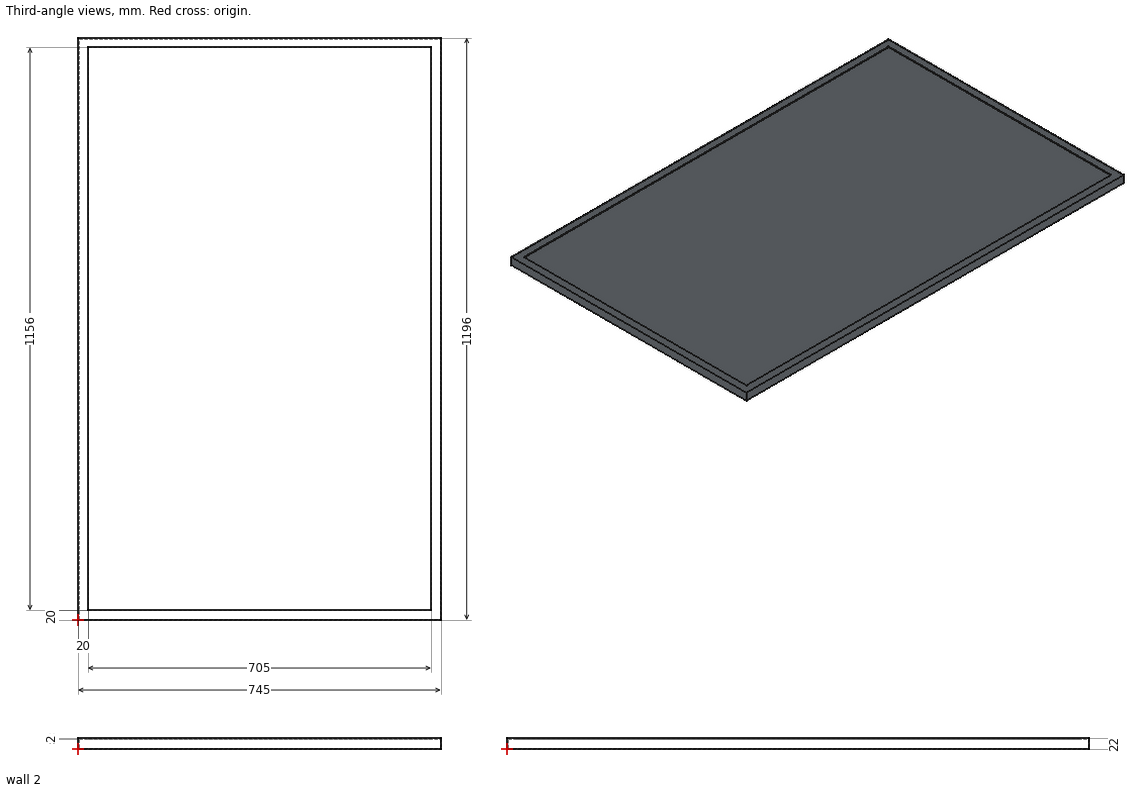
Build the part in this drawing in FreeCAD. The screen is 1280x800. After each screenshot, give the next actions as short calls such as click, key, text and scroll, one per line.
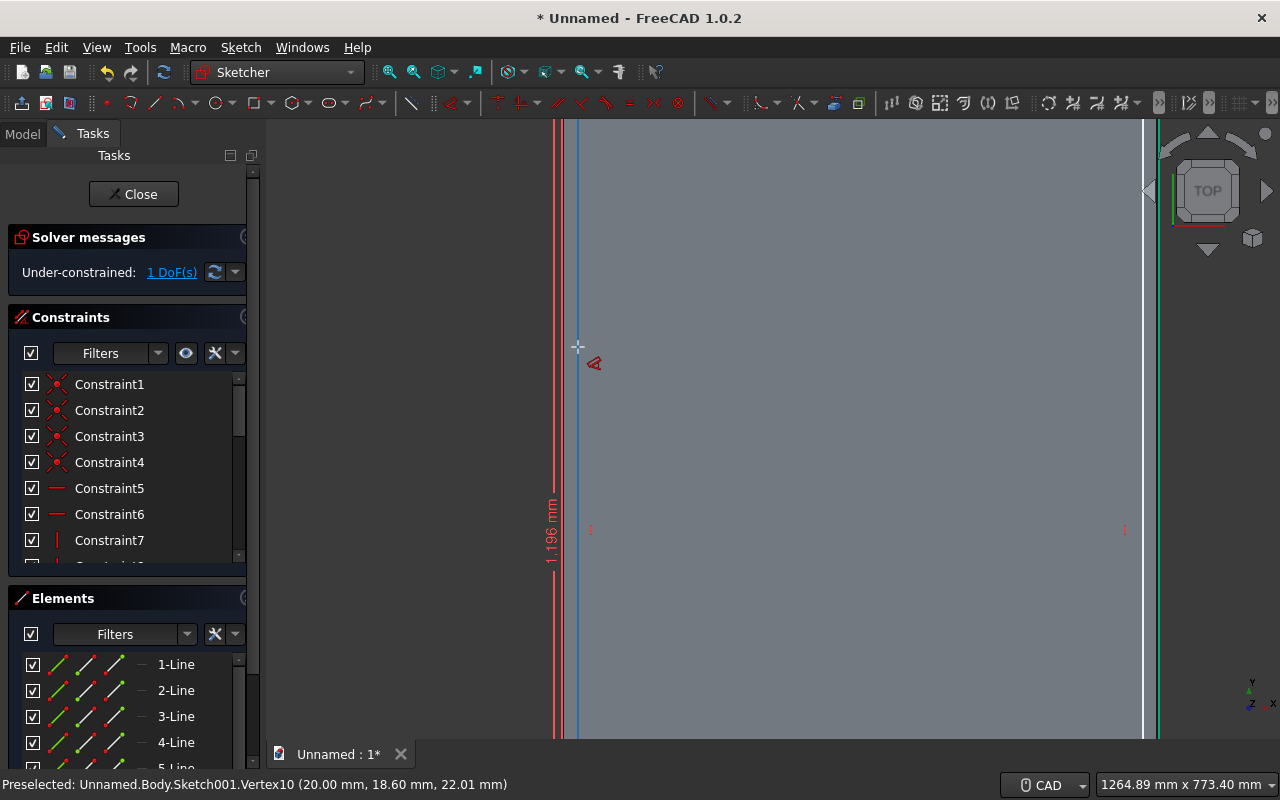
click(578, 347)
click(544, 429)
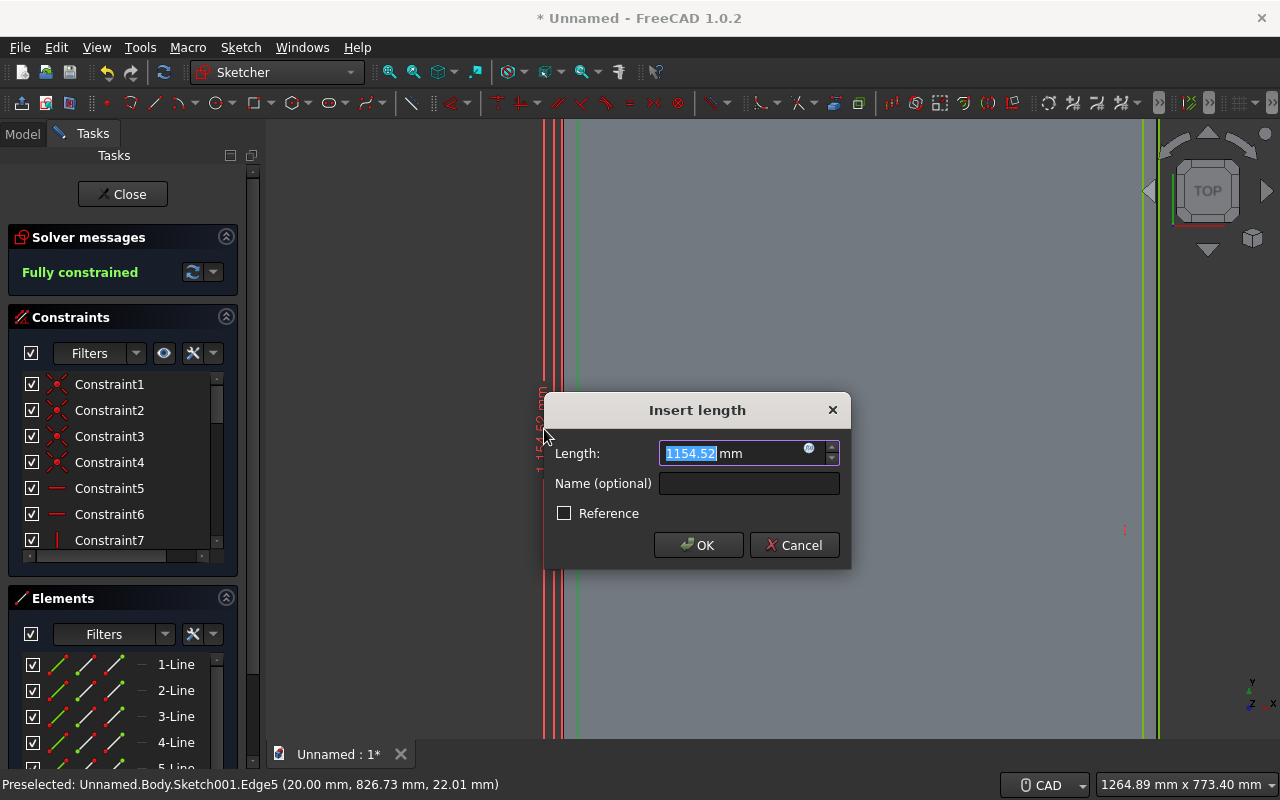
text(1156)
key(Return)
key(Escape)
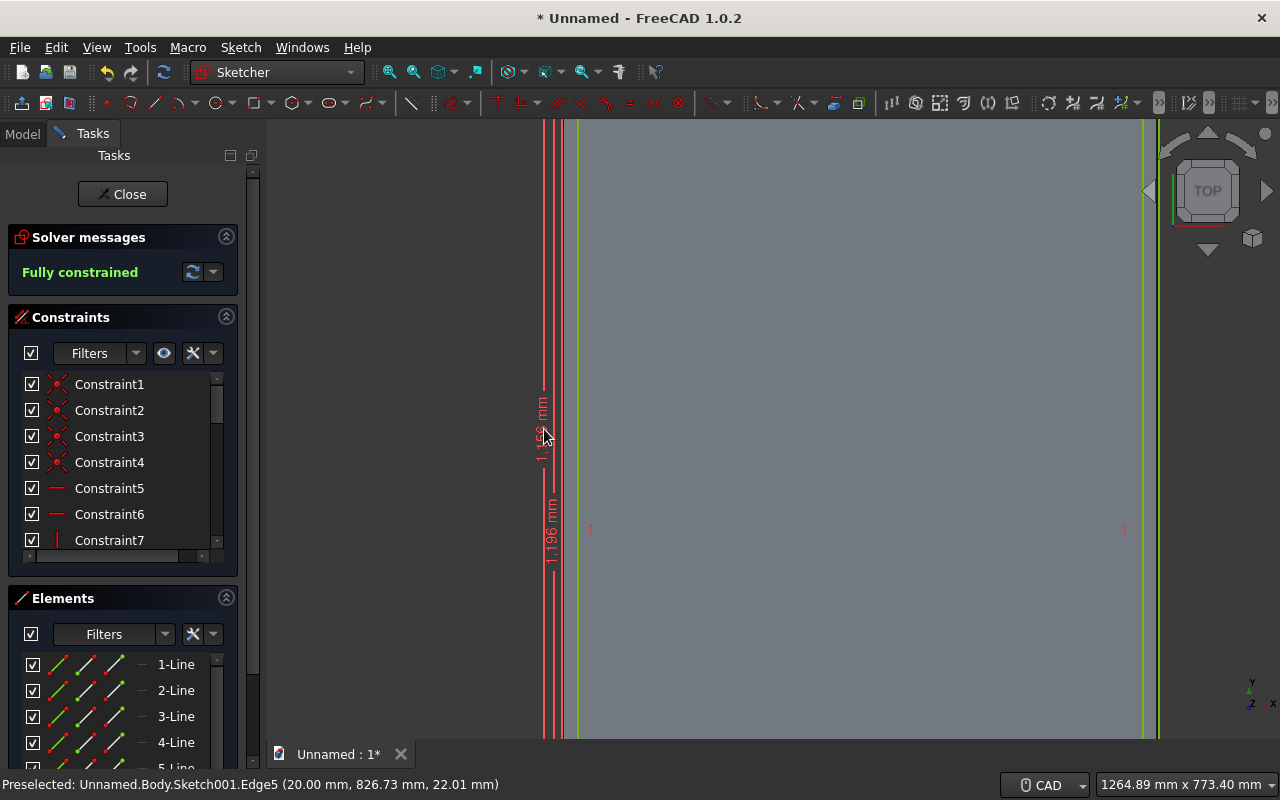
click(123, 194)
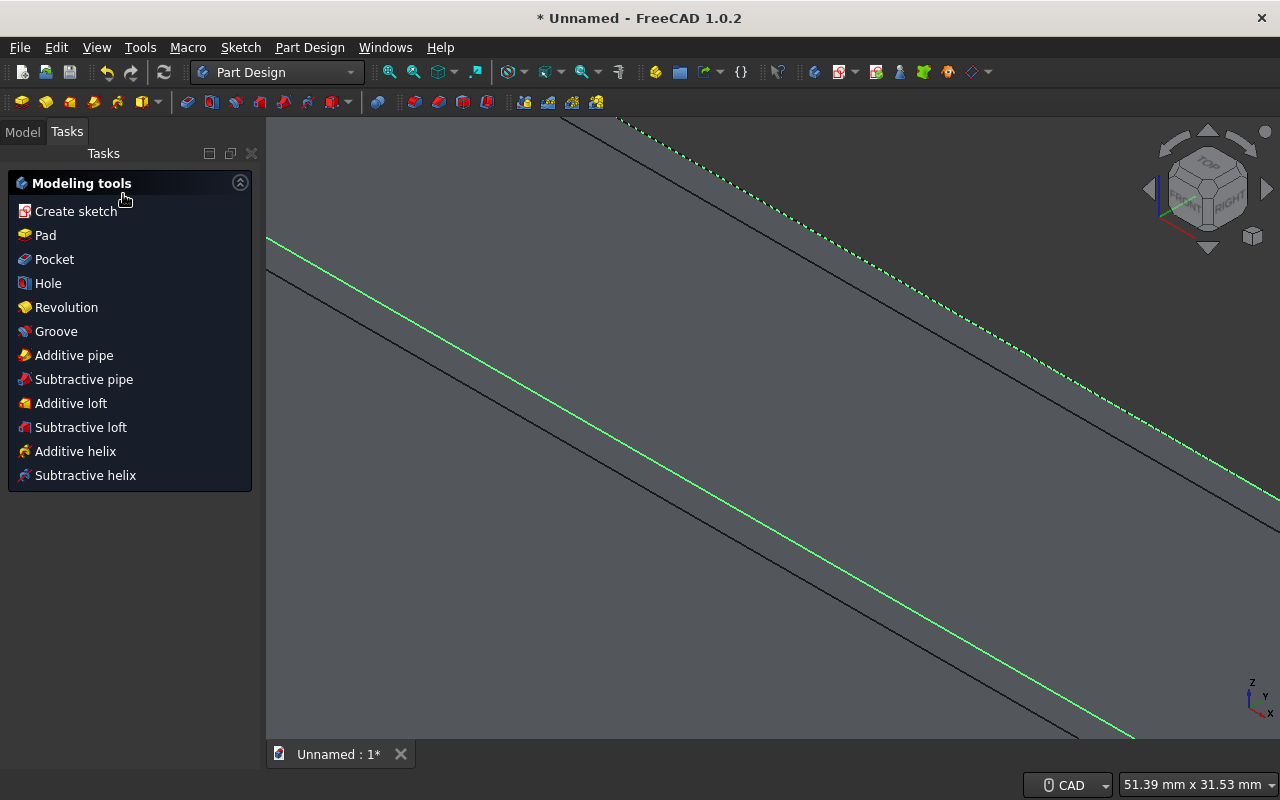
click(22, 102)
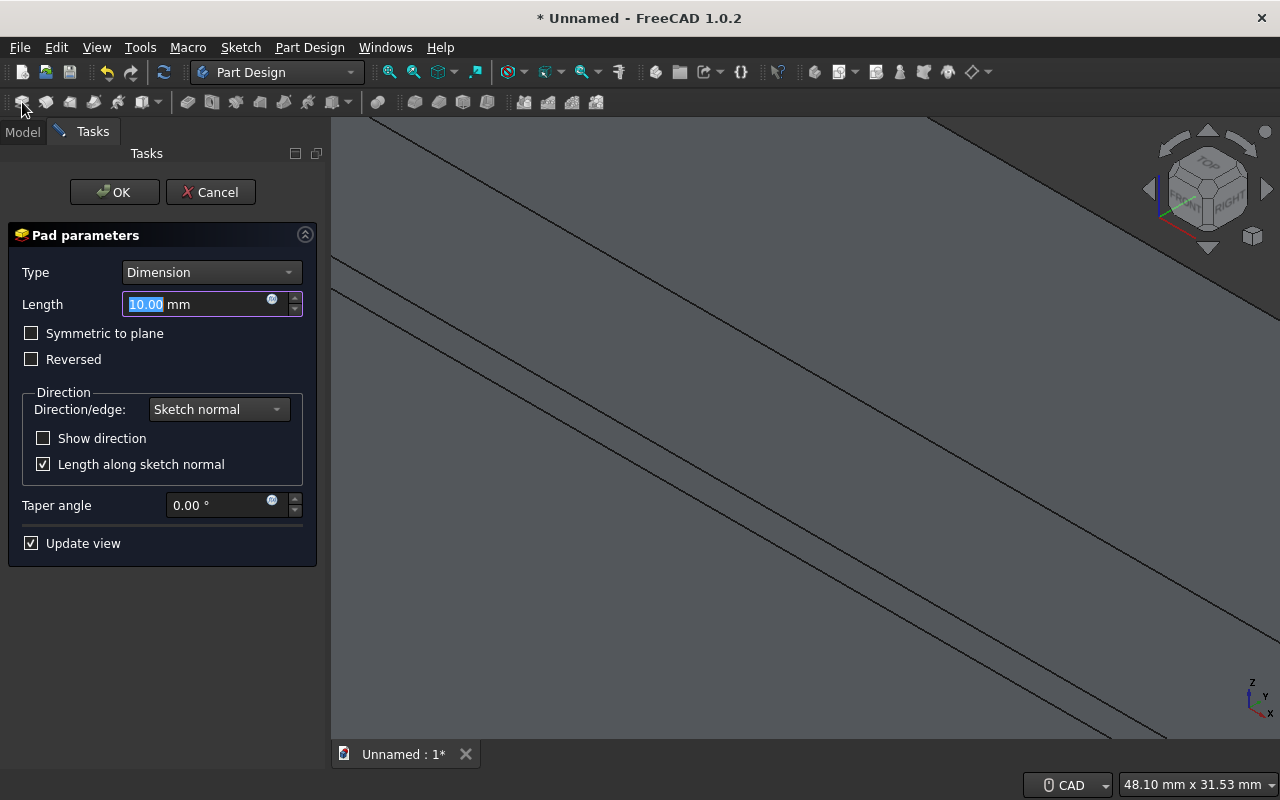
text(2)
key(Tab)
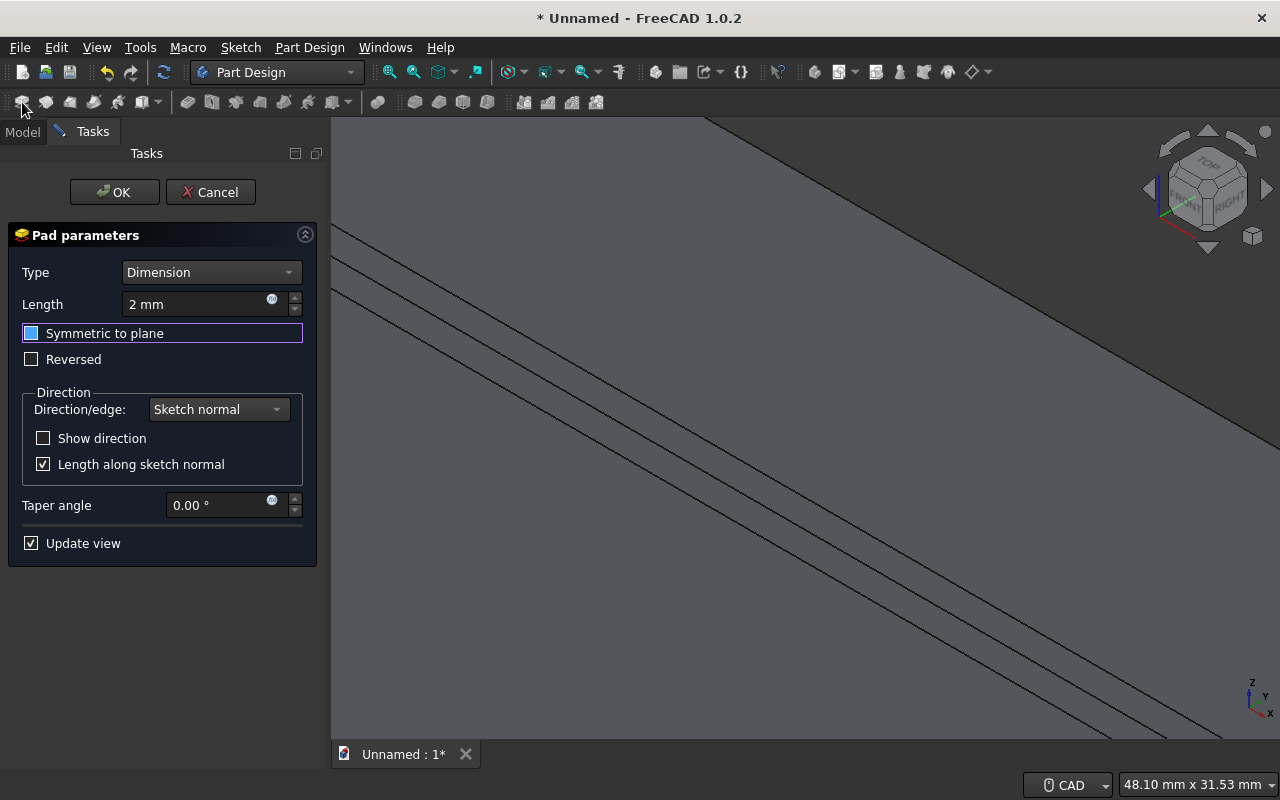
click(30, 359)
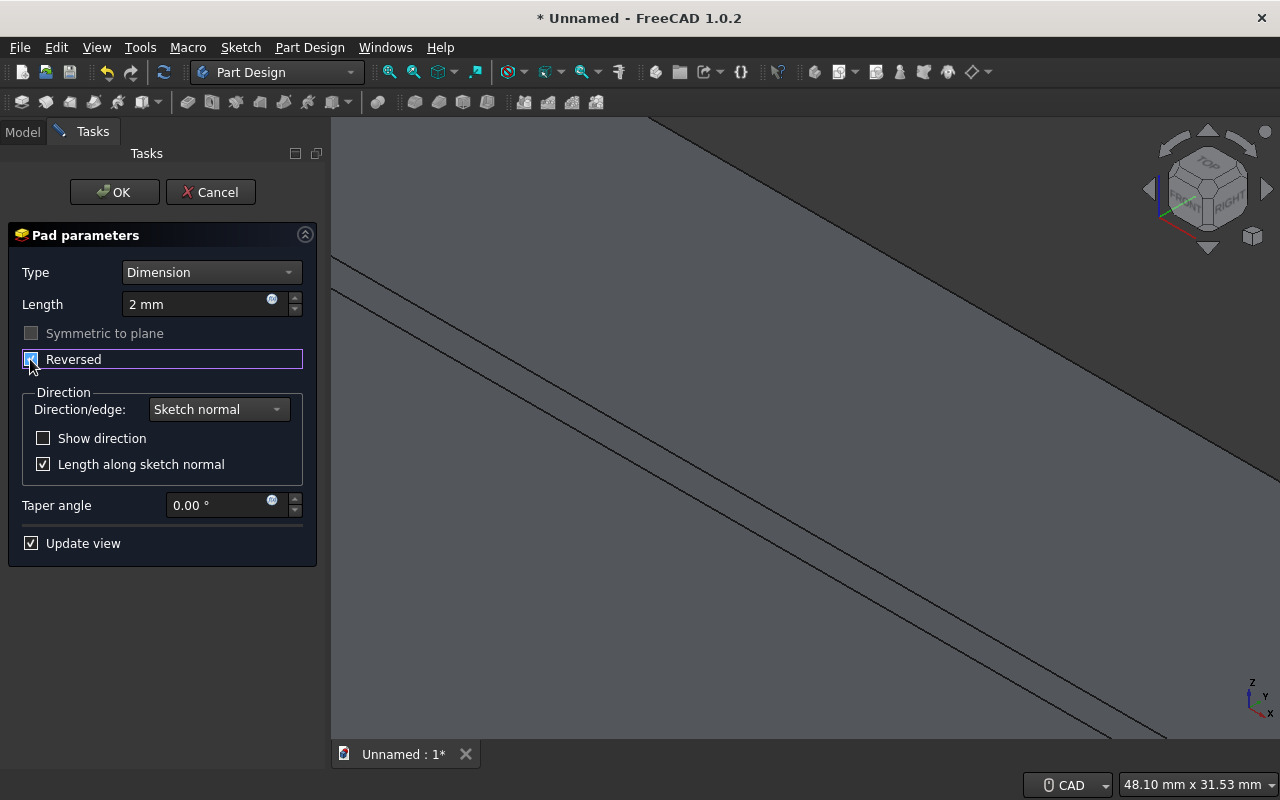
click(115, 192)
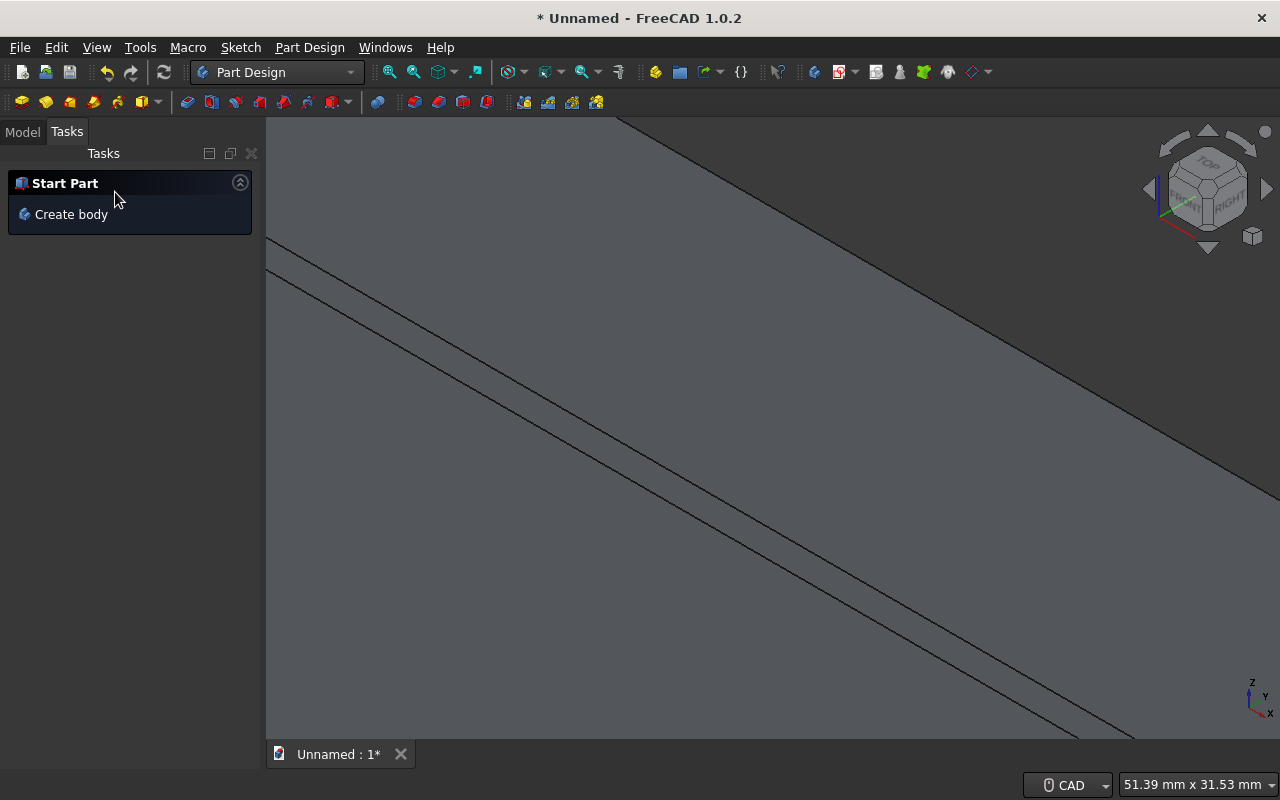
click(390, 72)